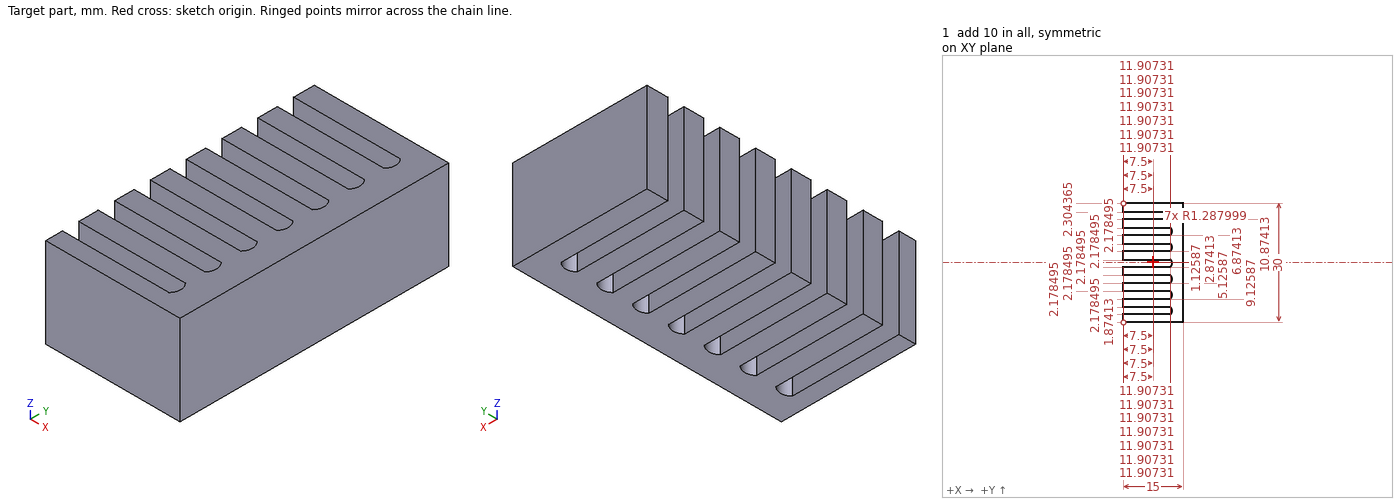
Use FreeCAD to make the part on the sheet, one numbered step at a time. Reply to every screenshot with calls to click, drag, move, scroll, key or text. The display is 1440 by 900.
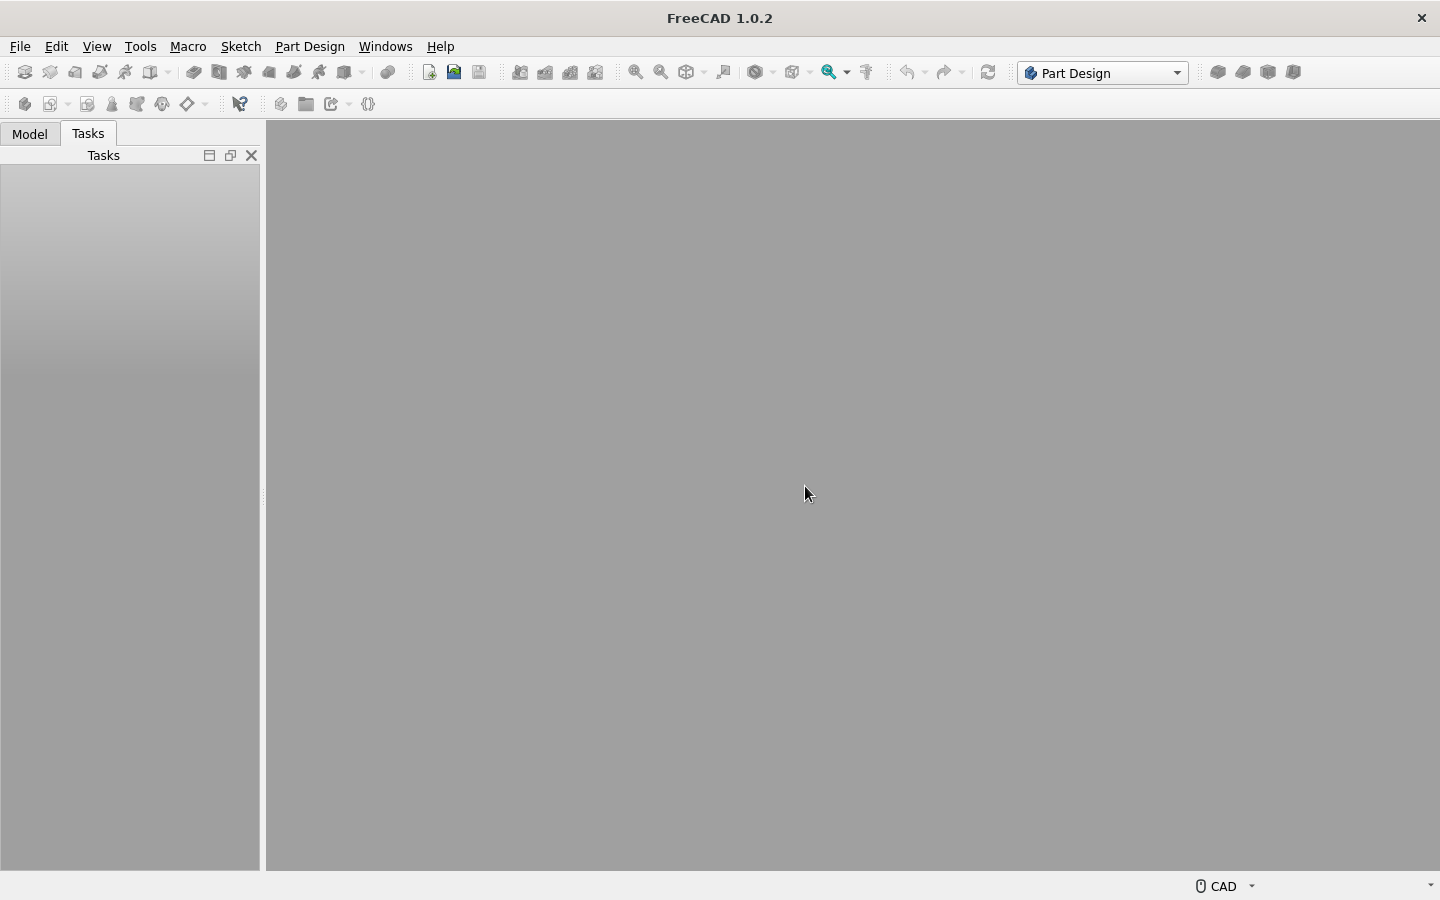
click(429, 72)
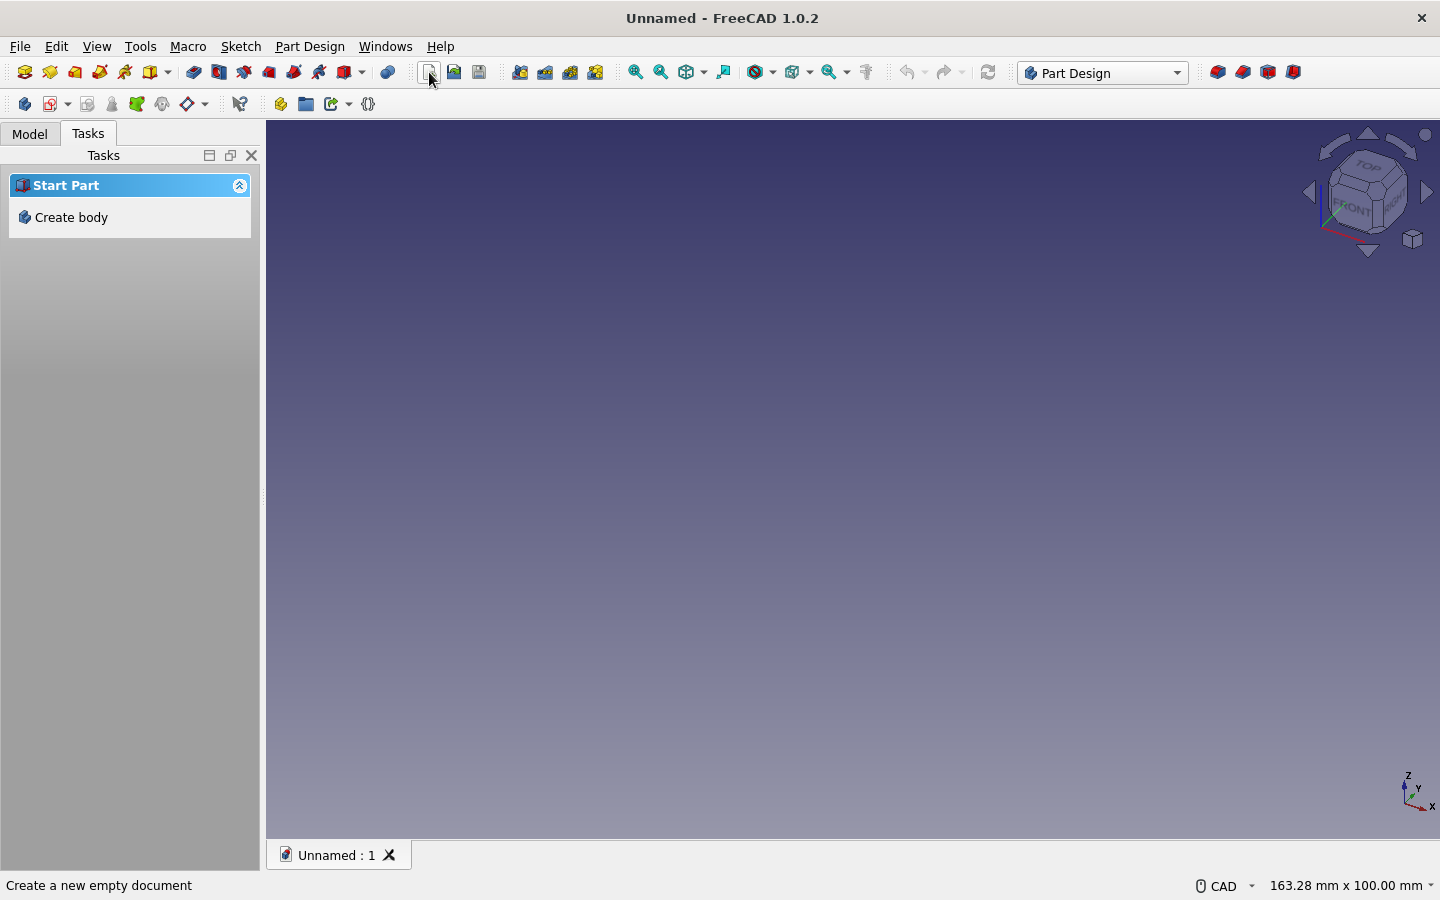
click(50, 104)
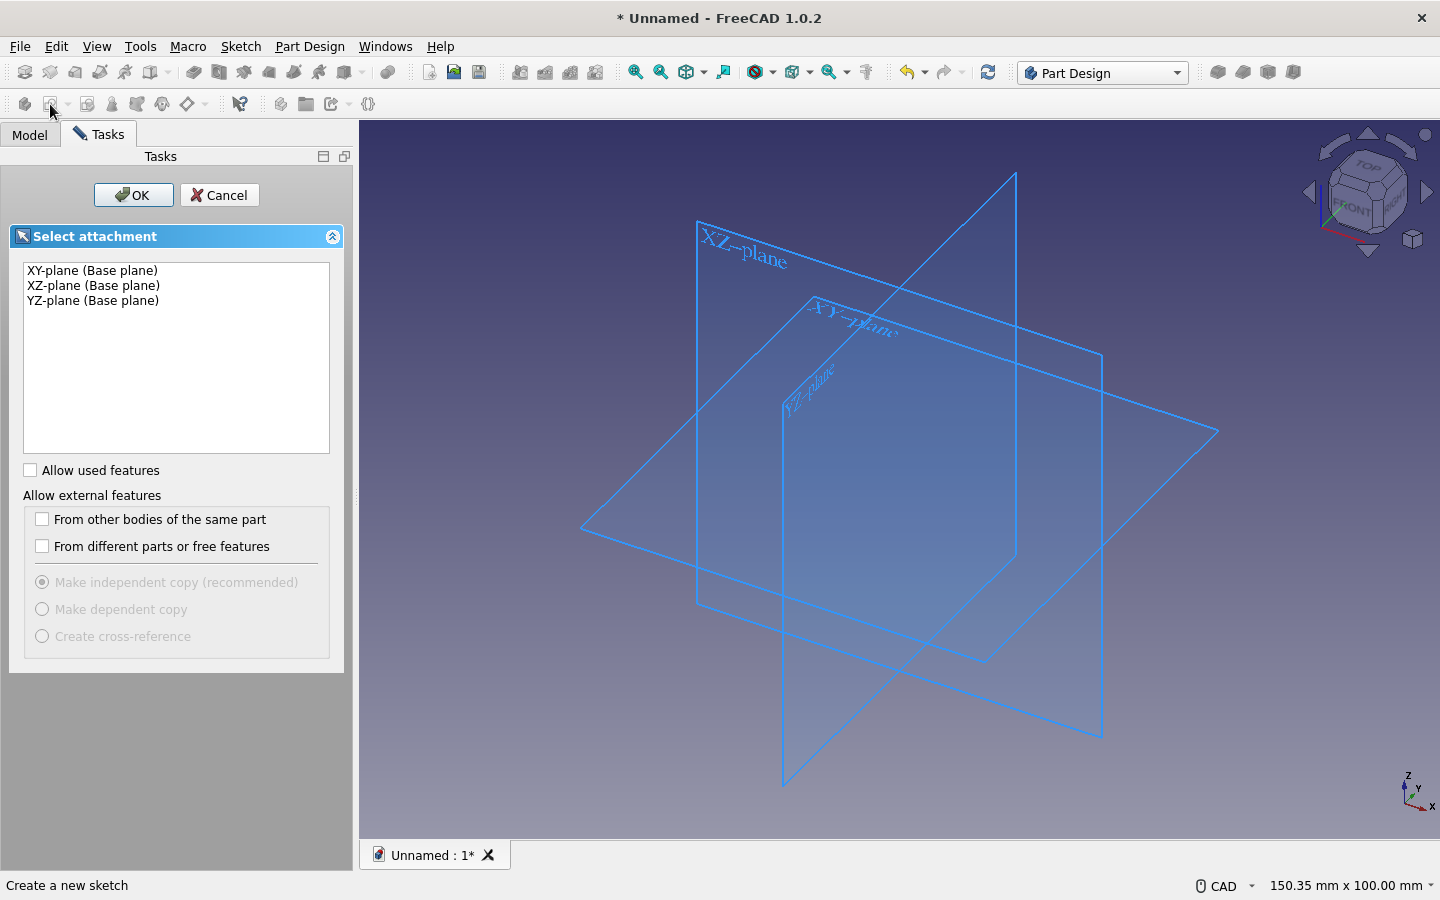
click(84, 270)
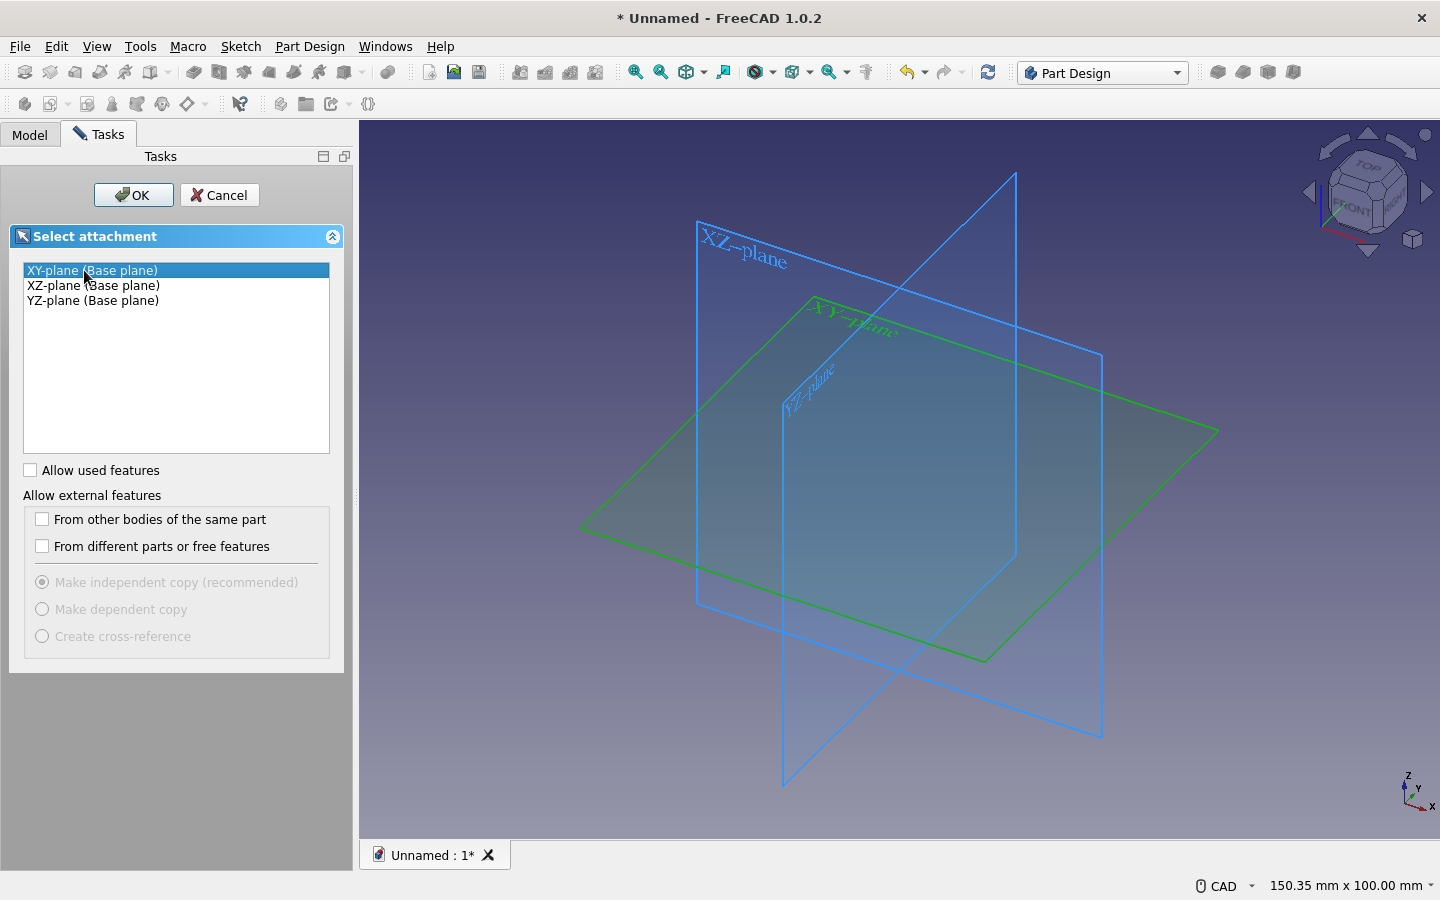
click(134, 195)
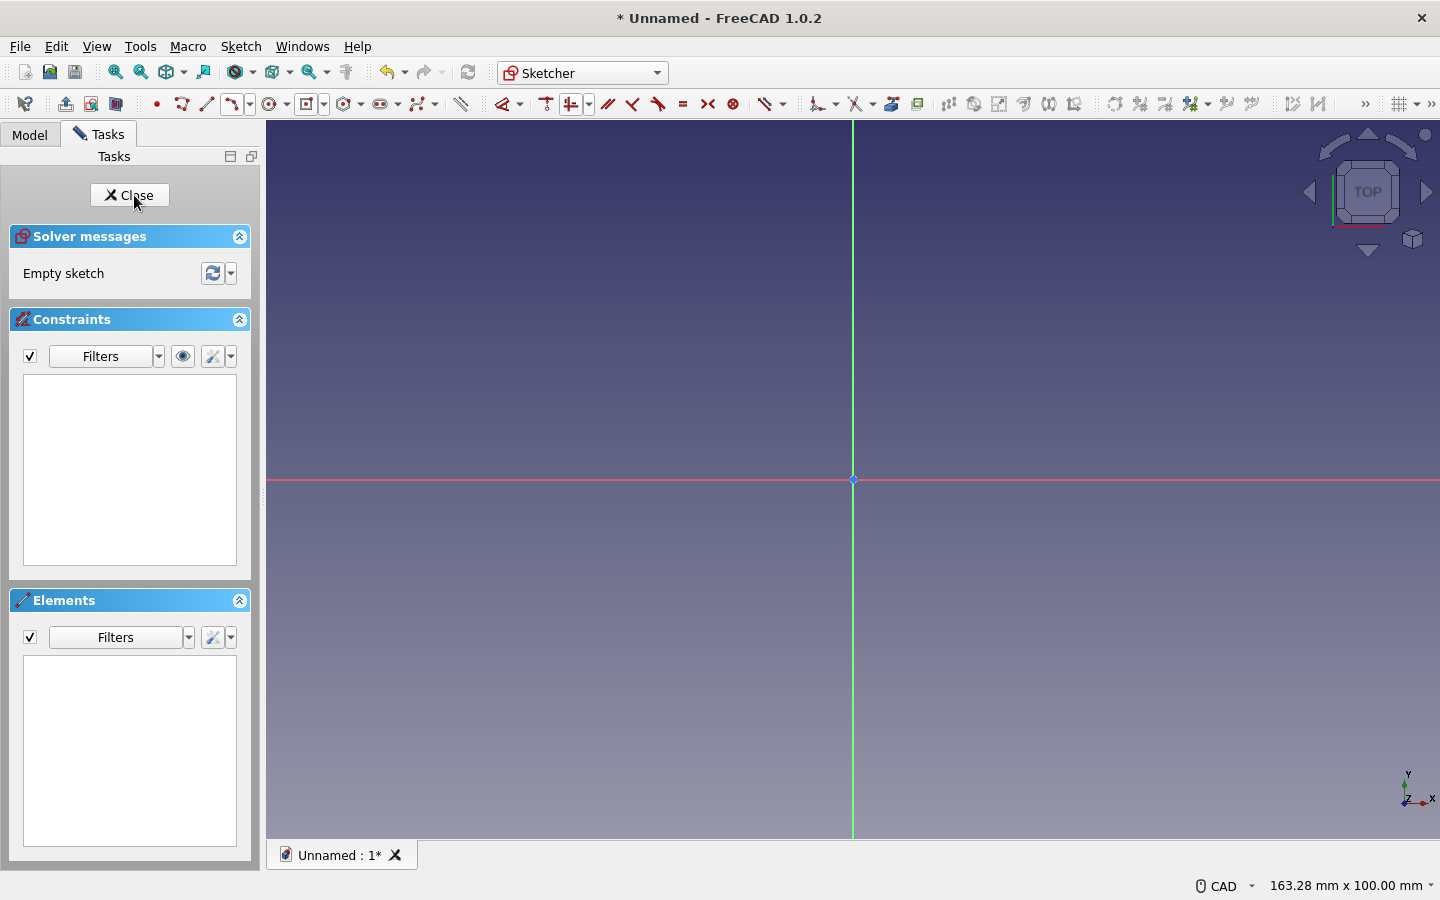
scroll(909, 480, up, 4)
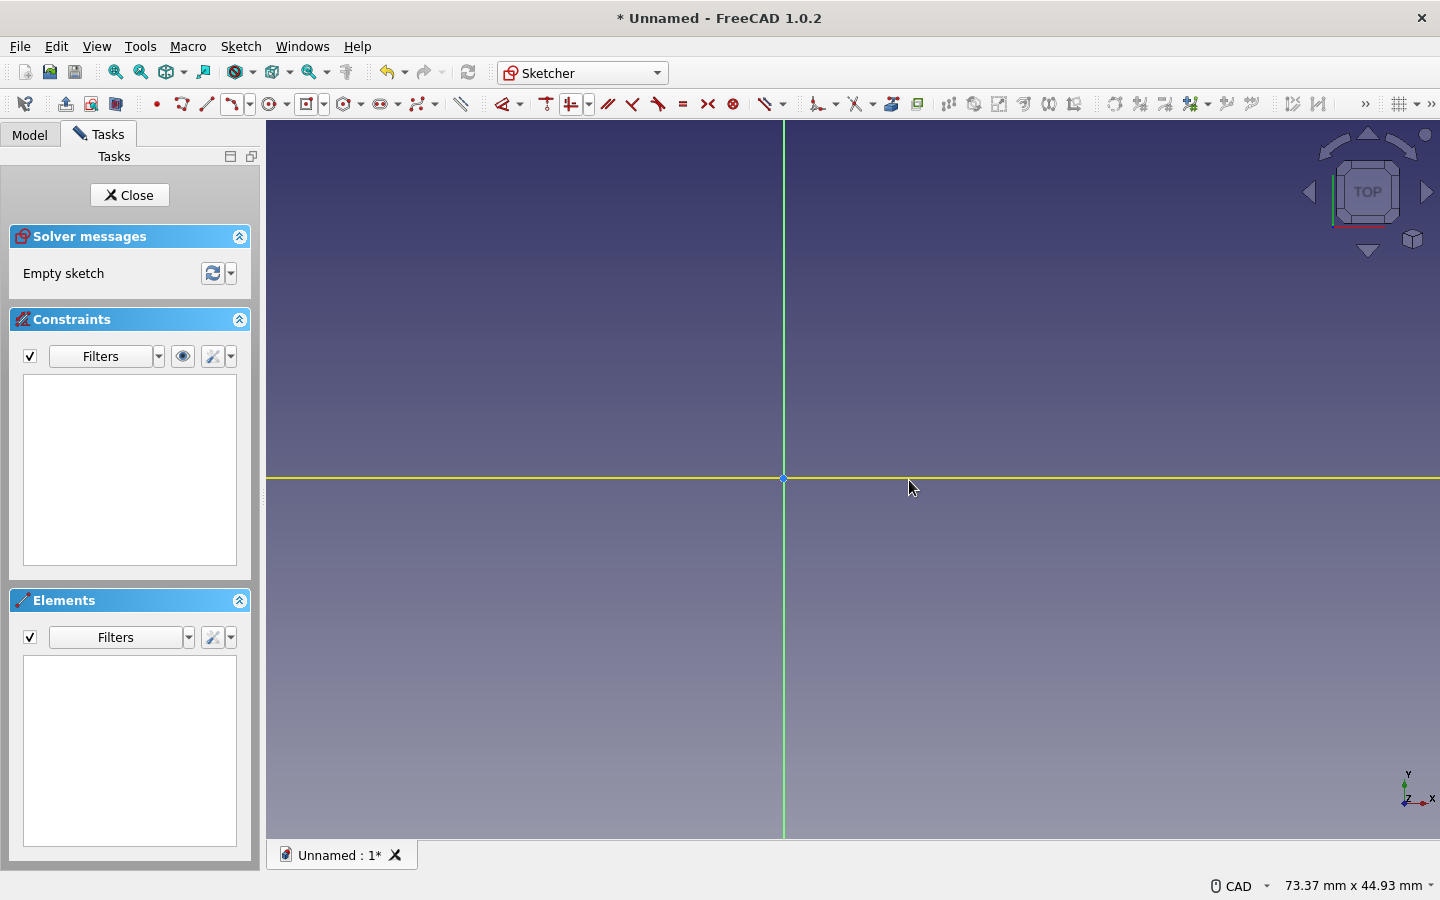
click(182, 104)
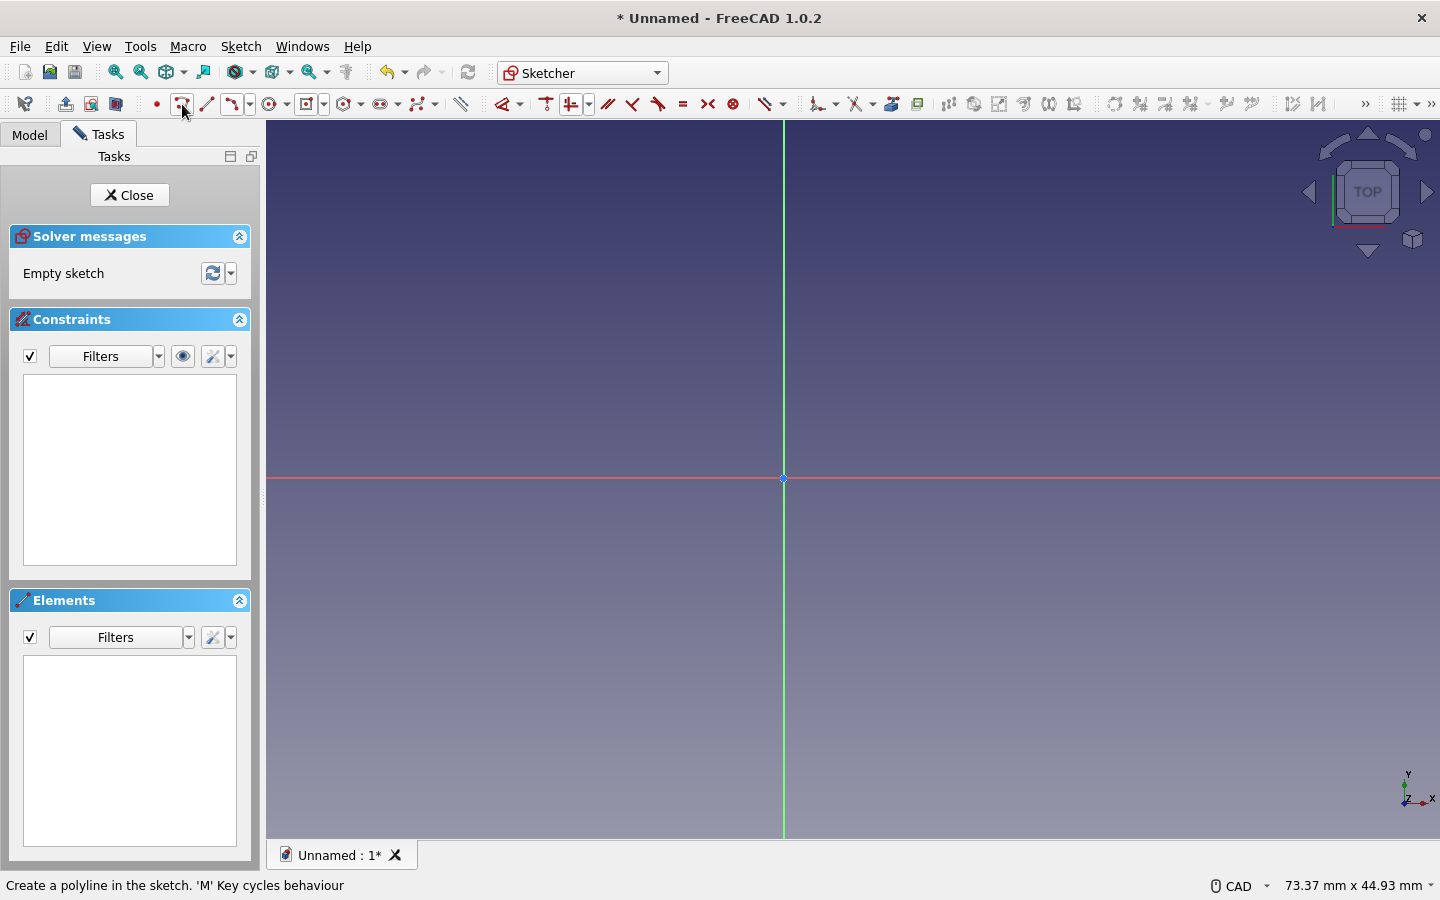
click(854, 304)
click(664, 304)
click(664, 339)
click(854, 339)
right_click(854, 339)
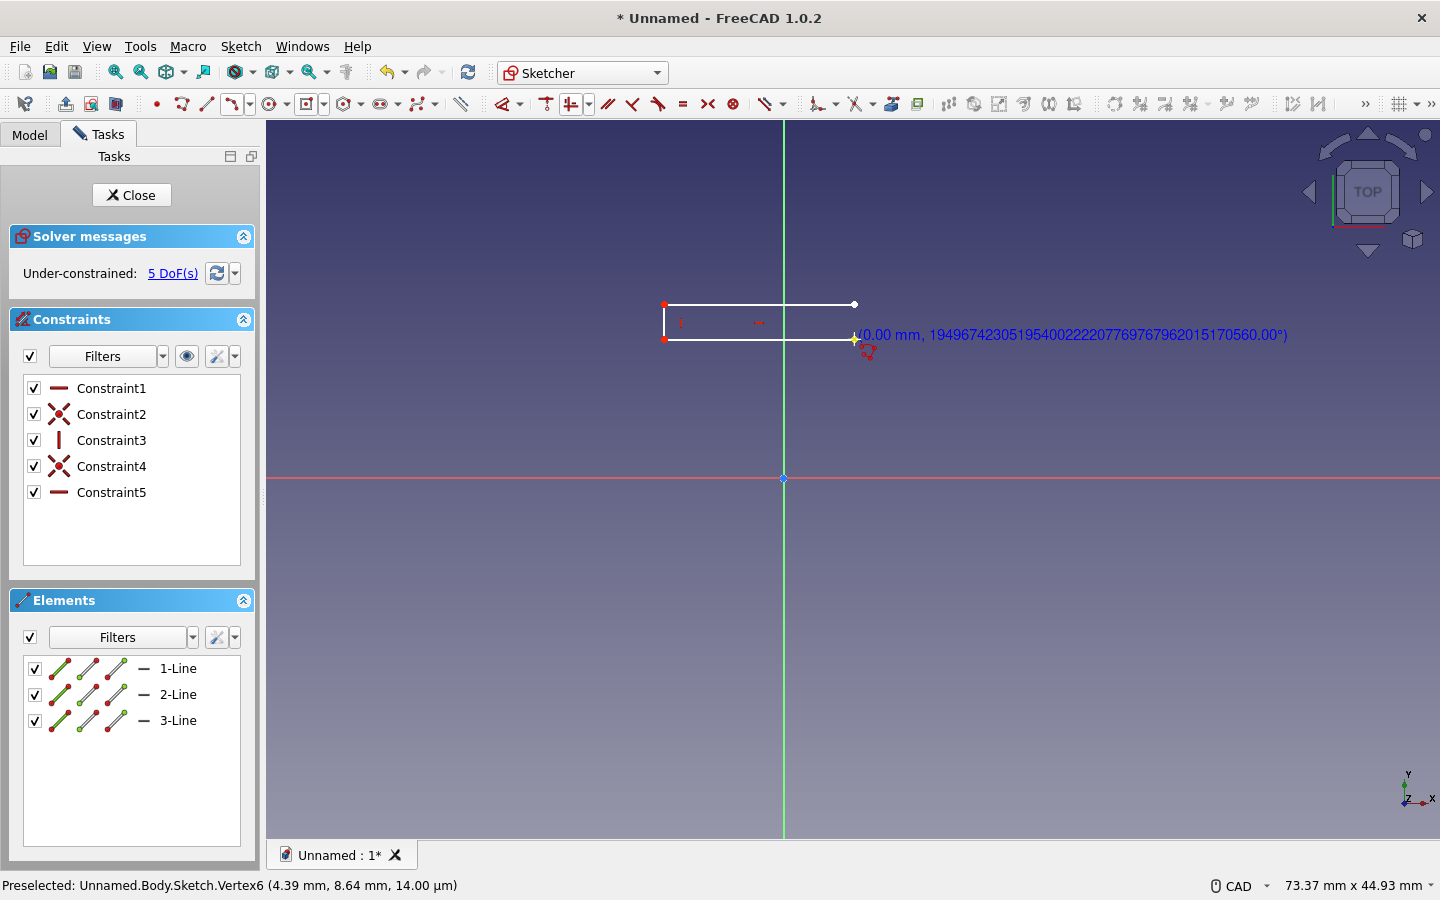
click(854, 368)
click(664, 368)
click(664, 403)
click(854, 403)
right_click(854, 403)